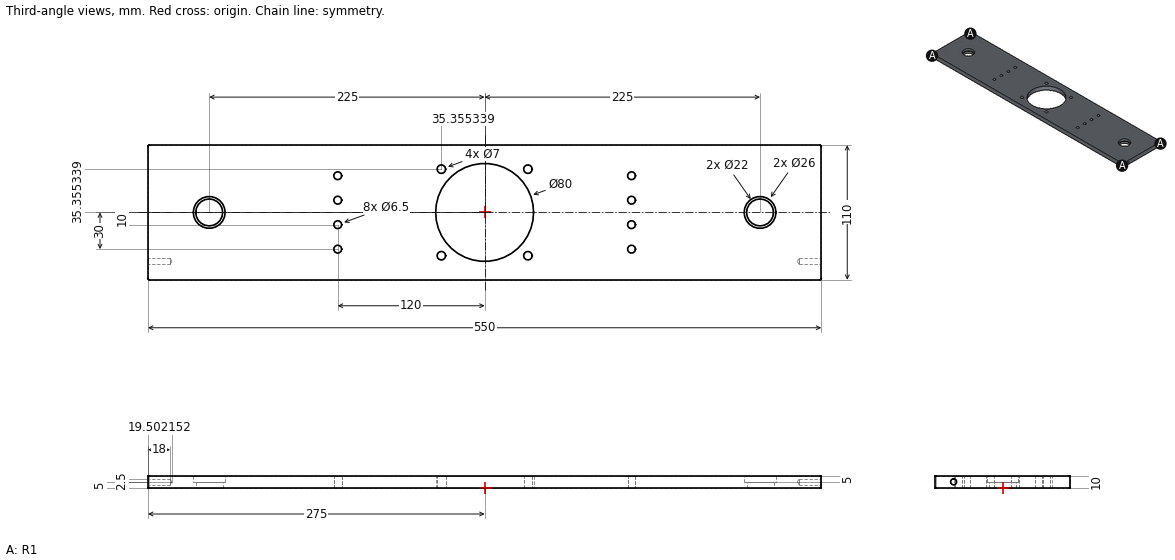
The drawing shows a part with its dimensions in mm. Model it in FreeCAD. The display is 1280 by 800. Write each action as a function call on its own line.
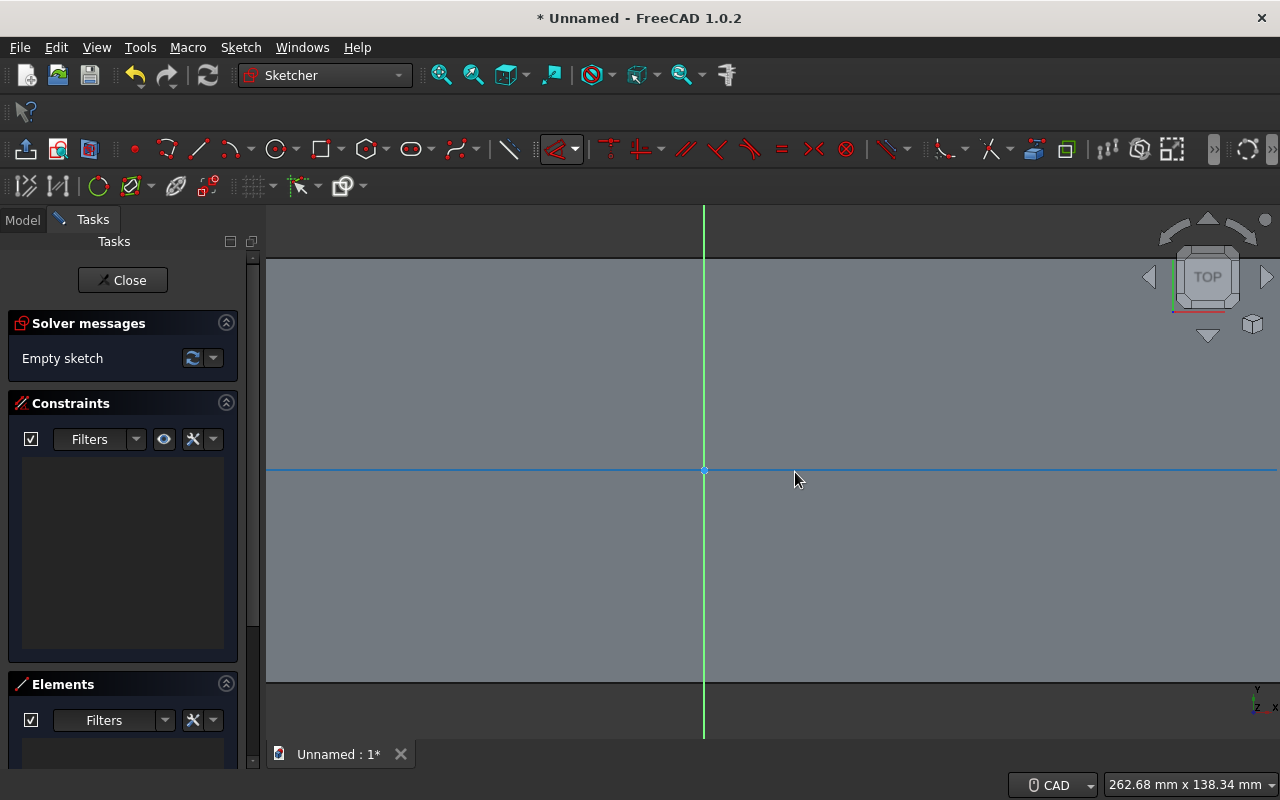
click(276, 150)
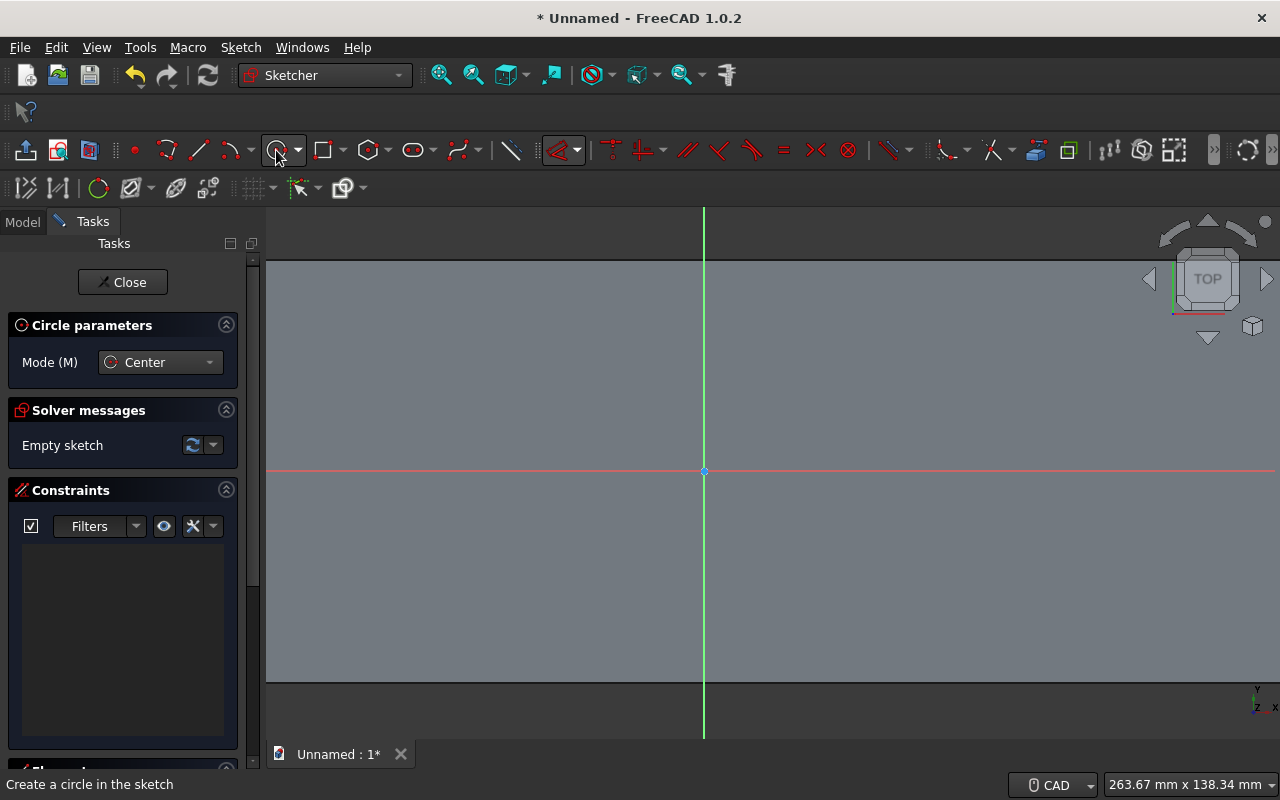
click(704, 471)
move(813, 363)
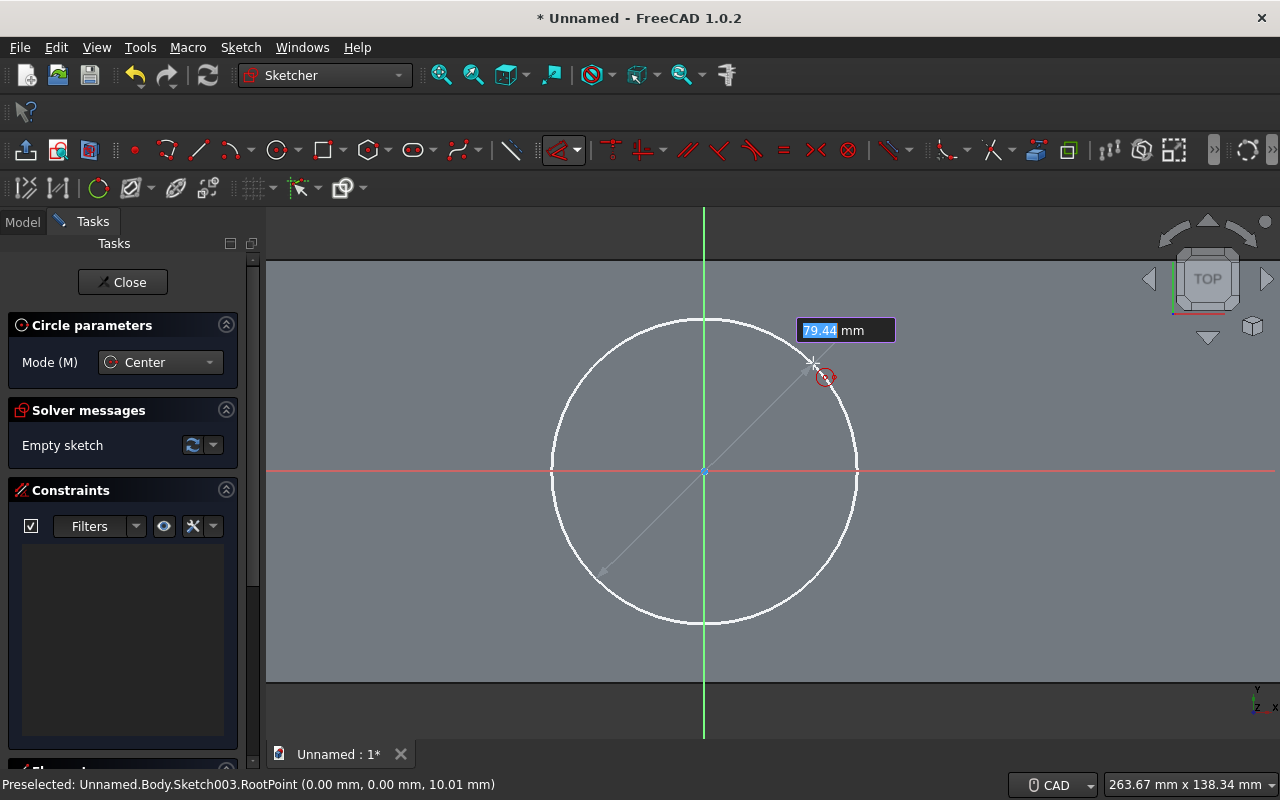
text(80)
key(Return)
key(Escape)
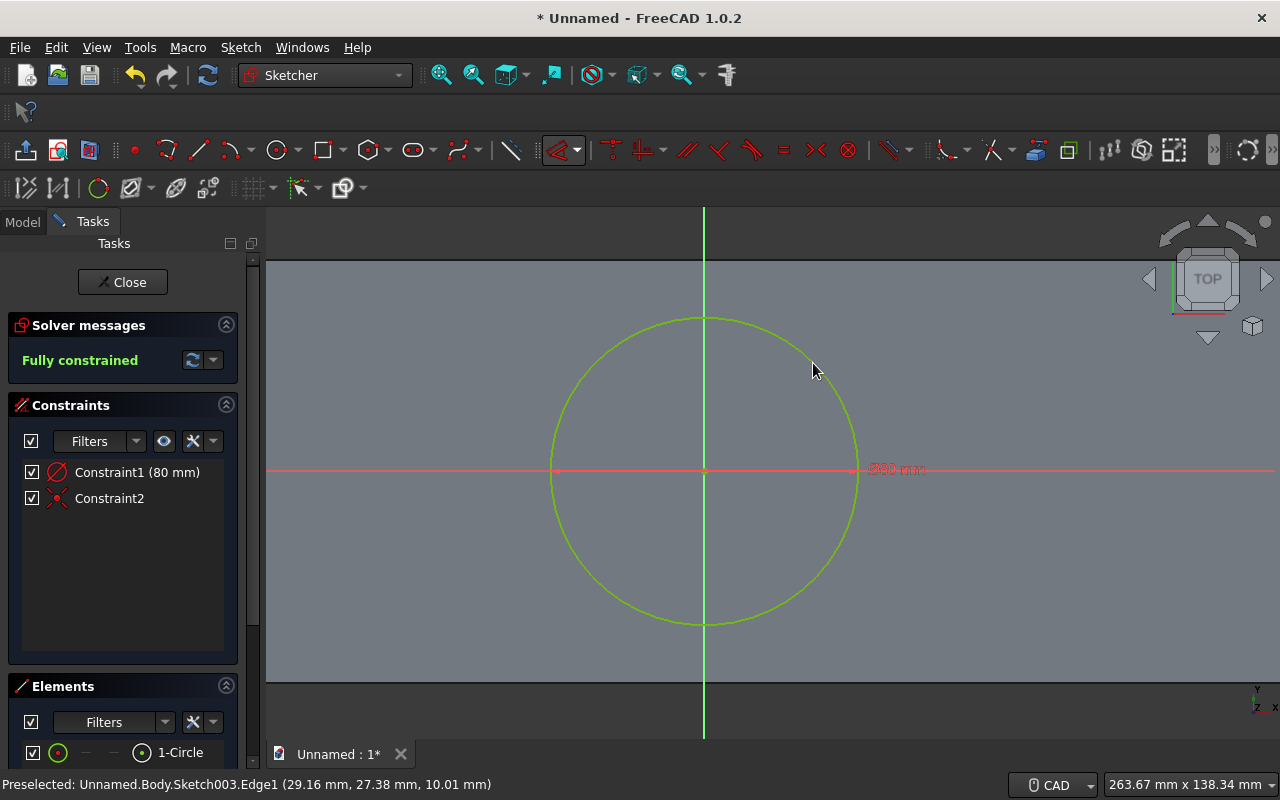
click(123, 282)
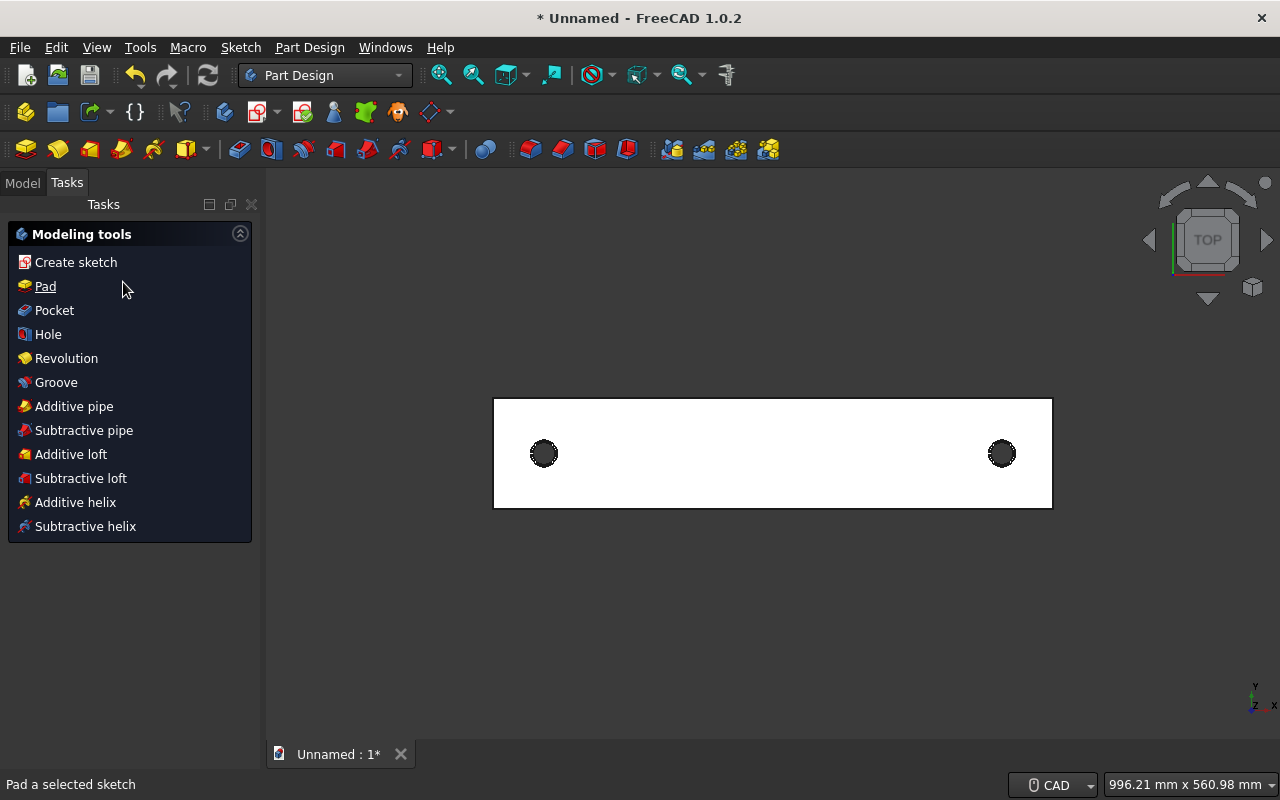
click(240, 150)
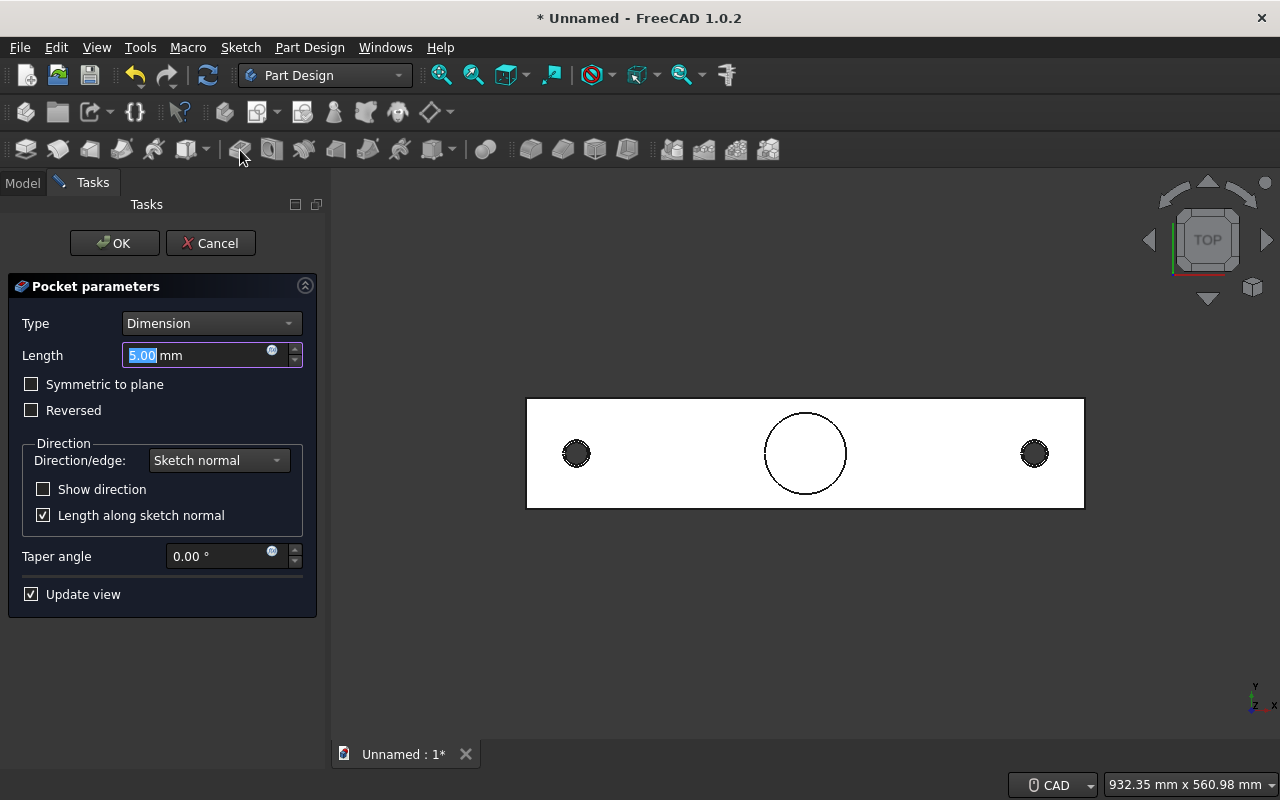
click(212, 324)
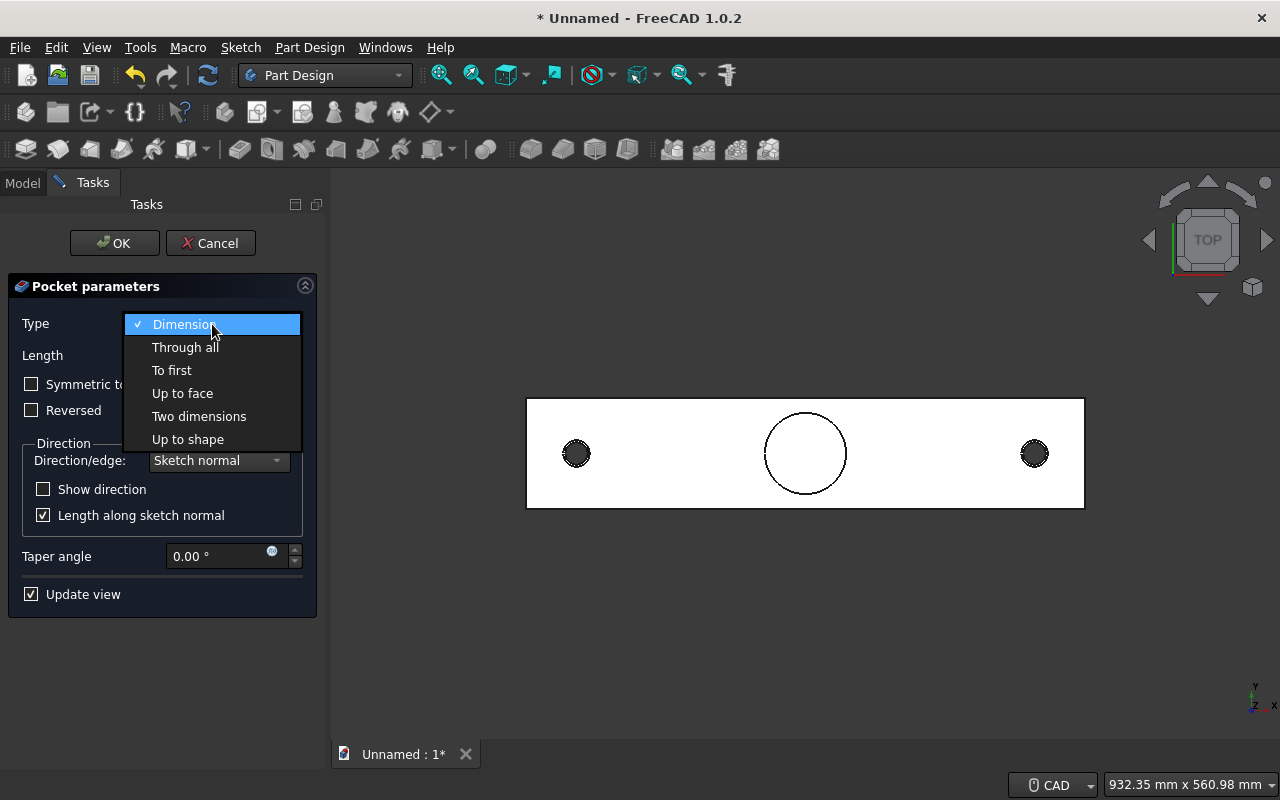
click(212, 348)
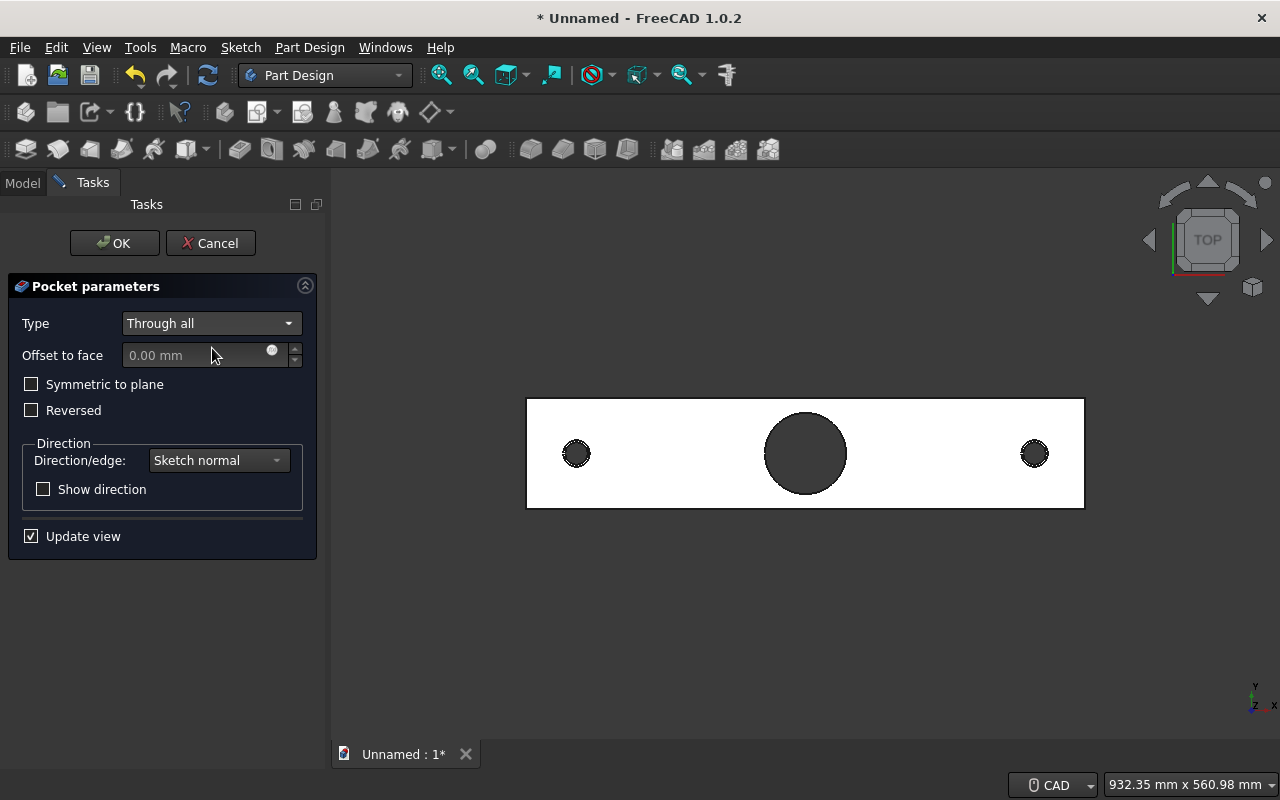
click(115, 243)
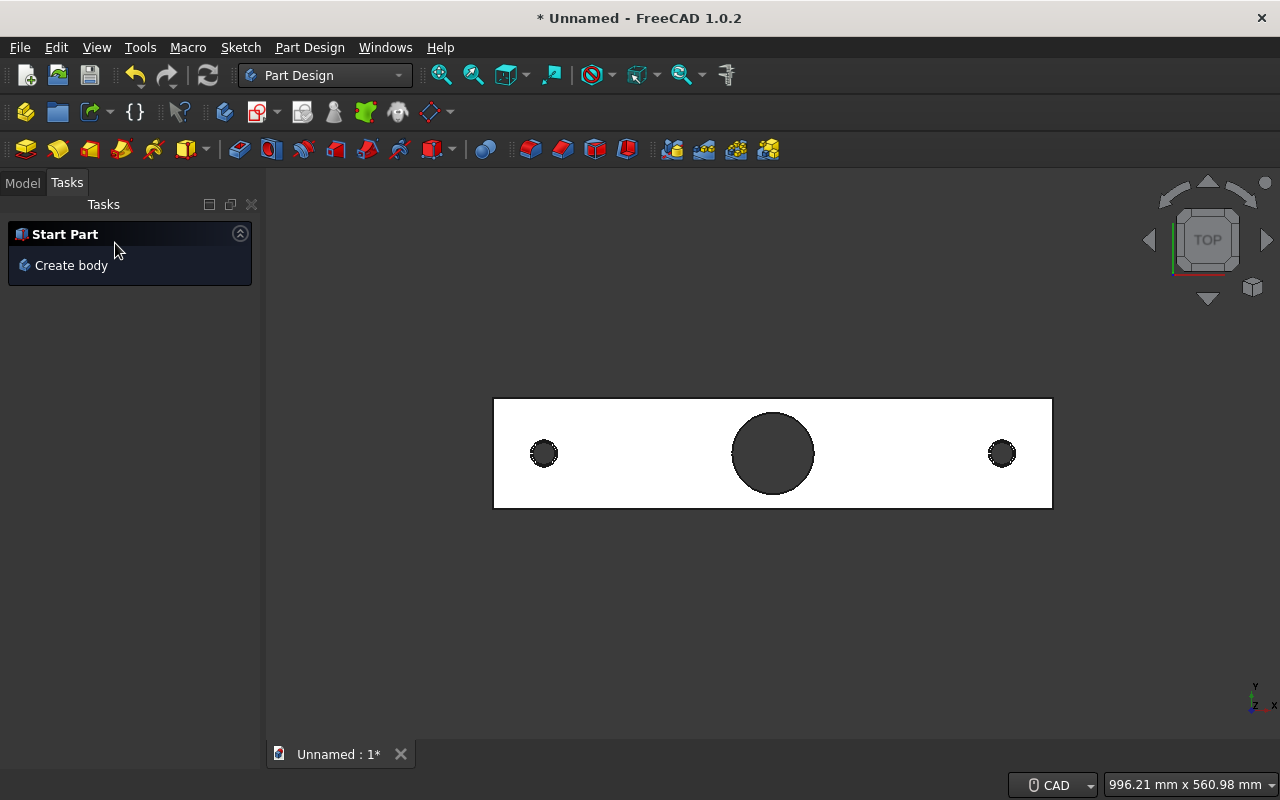
click(613, 452)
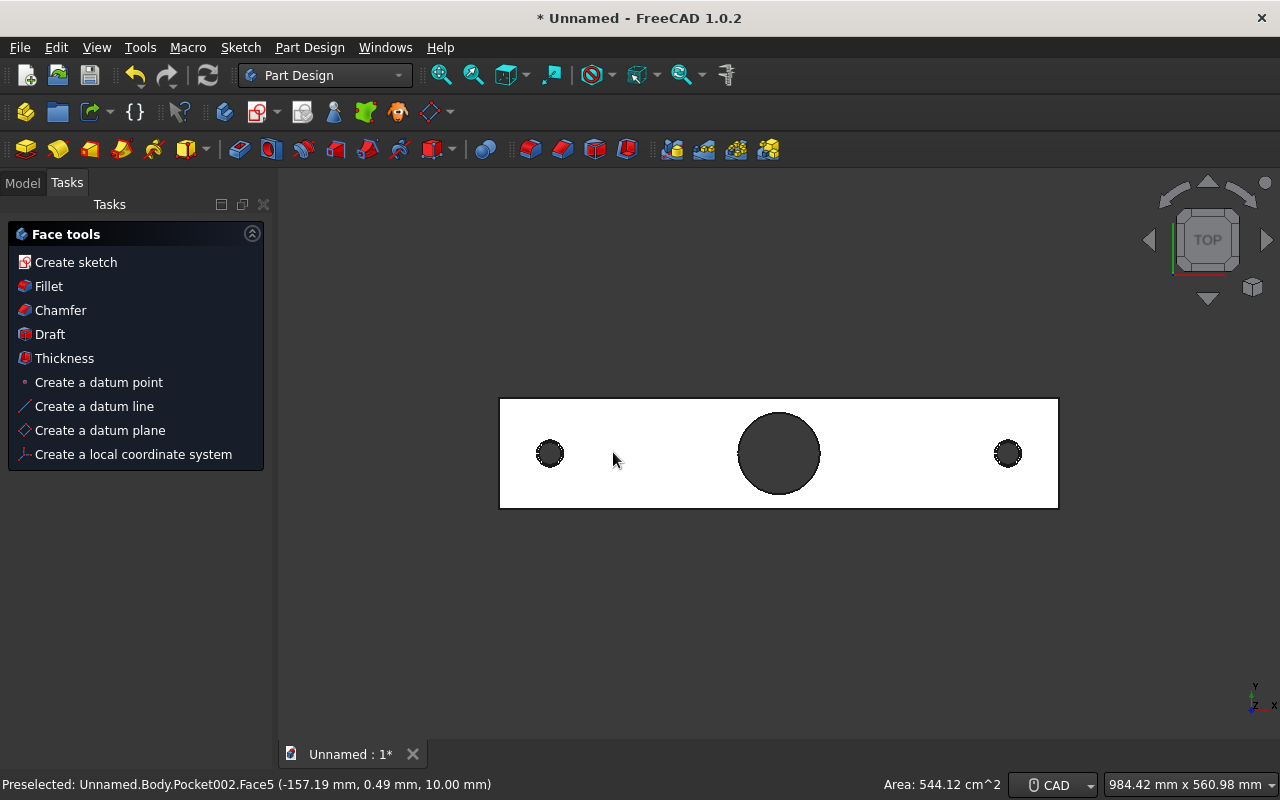
click(258, 112)